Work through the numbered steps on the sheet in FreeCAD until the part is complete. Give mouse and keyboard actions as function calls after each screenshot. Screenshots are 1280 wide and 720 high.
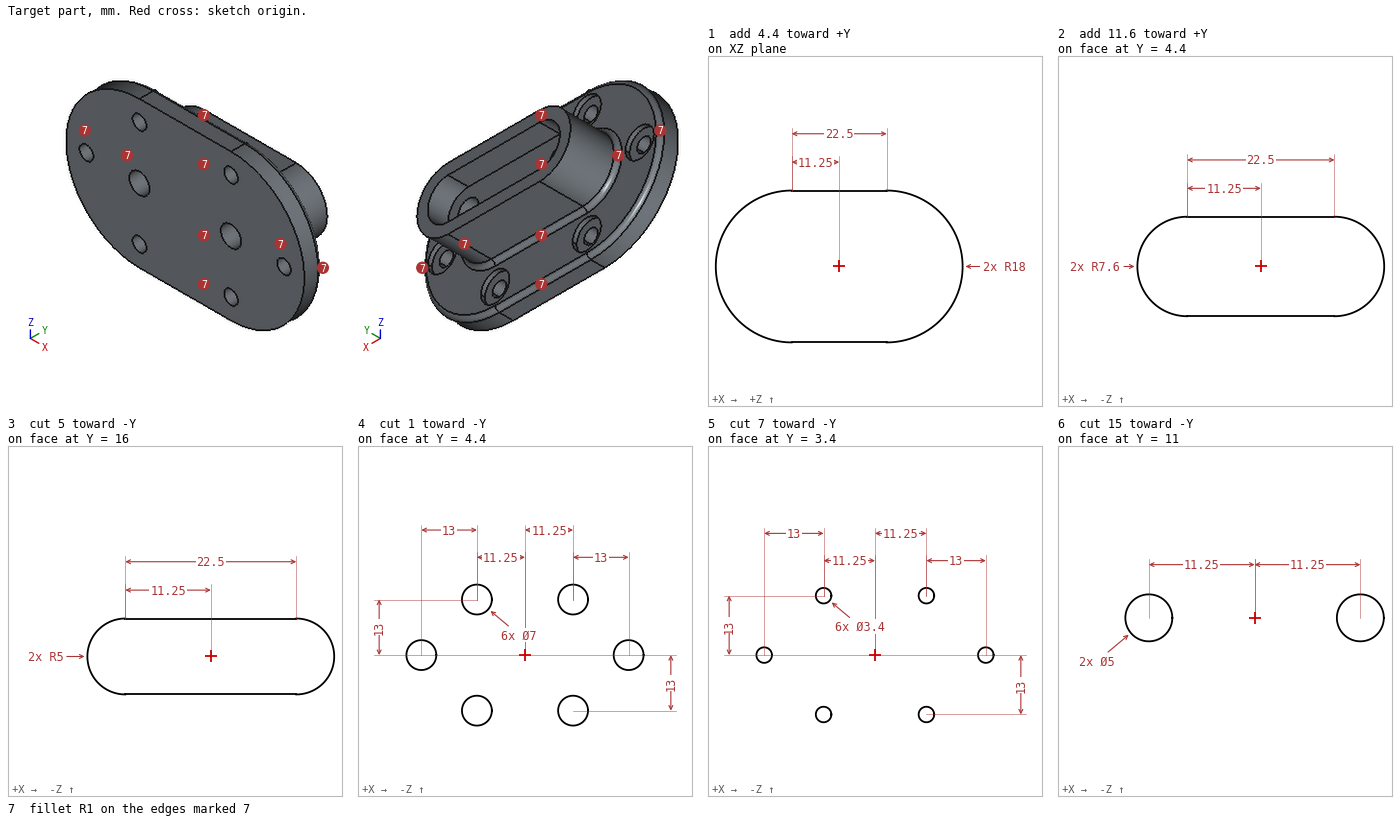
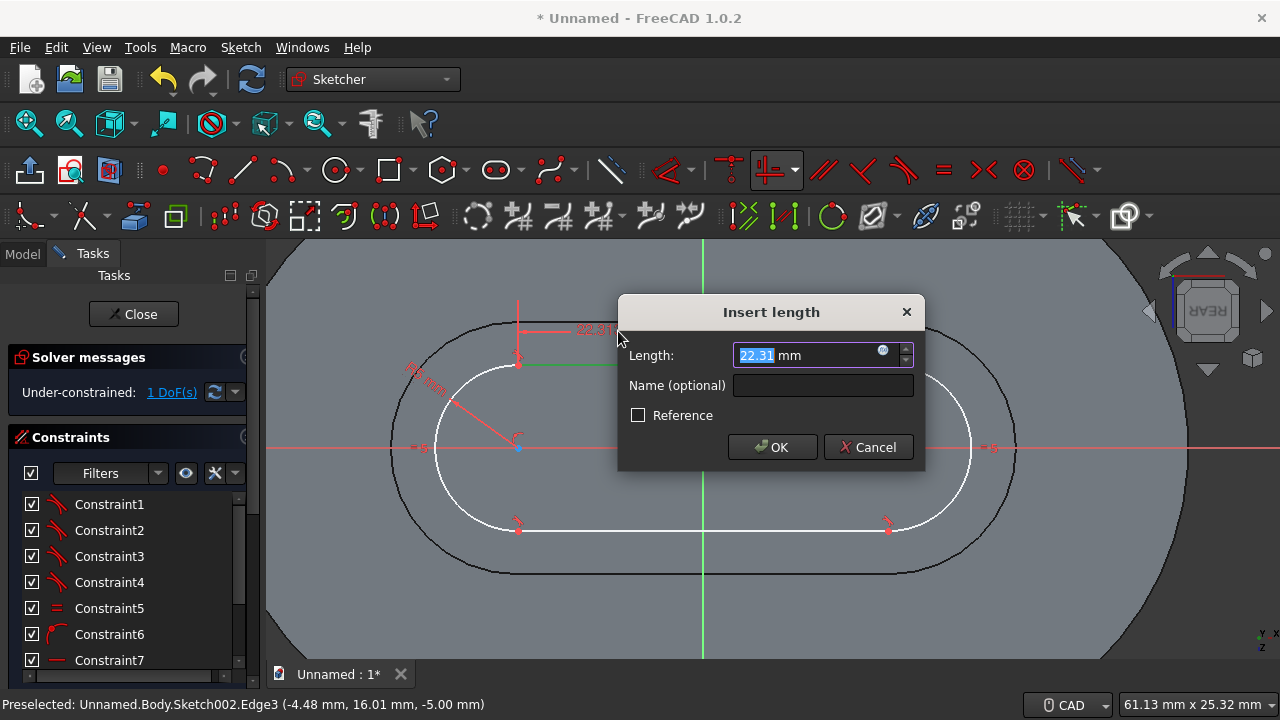
text(22.5)
key(Return)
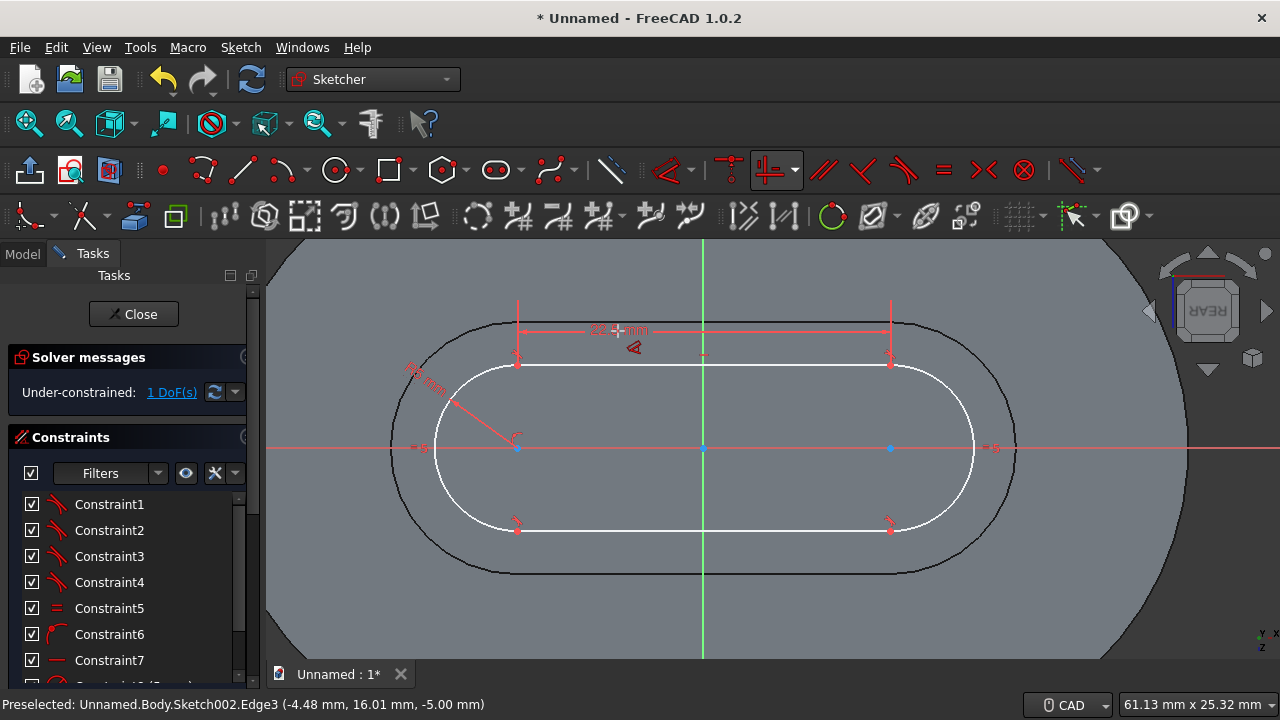
click(518, 365)
click(546, 331)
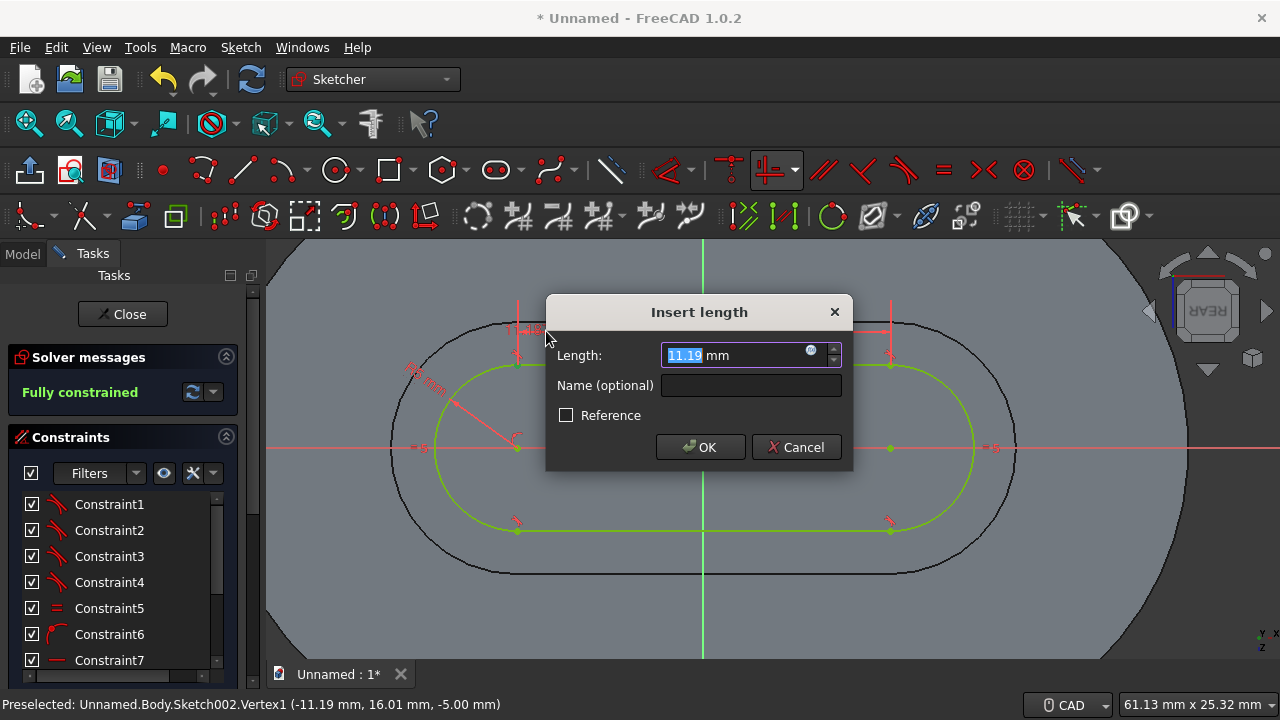
text(11.25)
key(Return)
key(Escape)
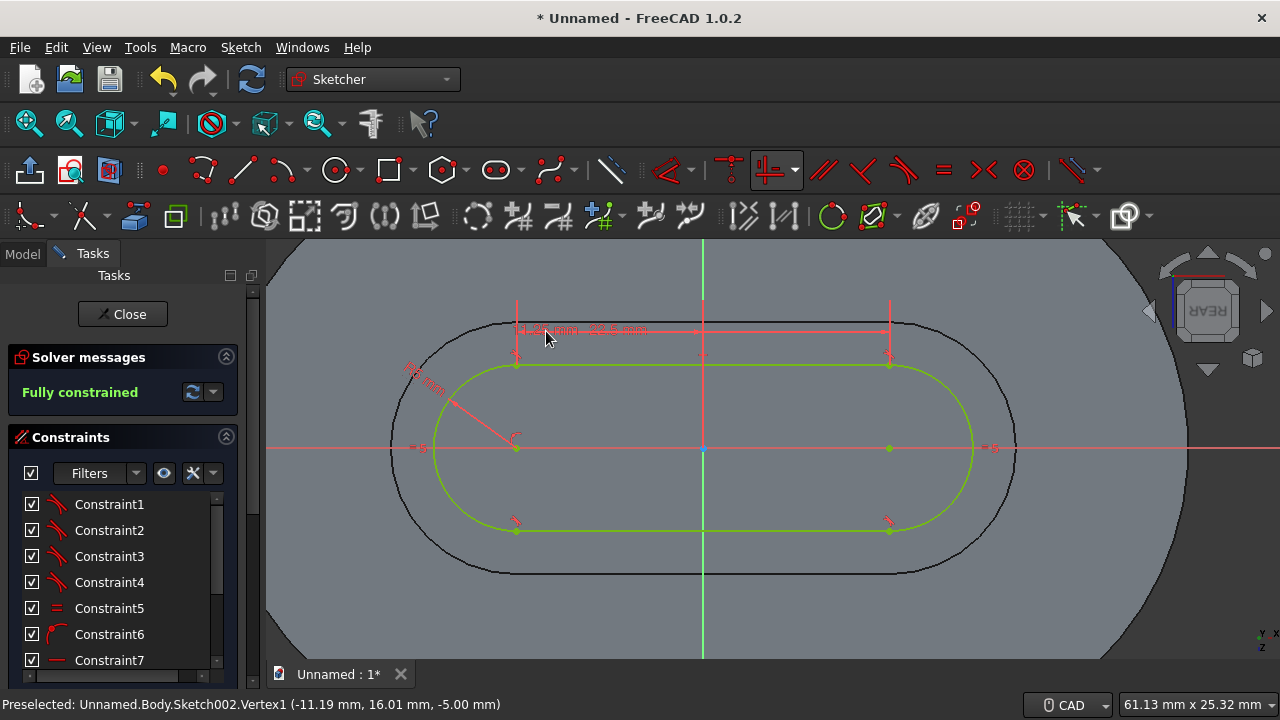
click(123, 314)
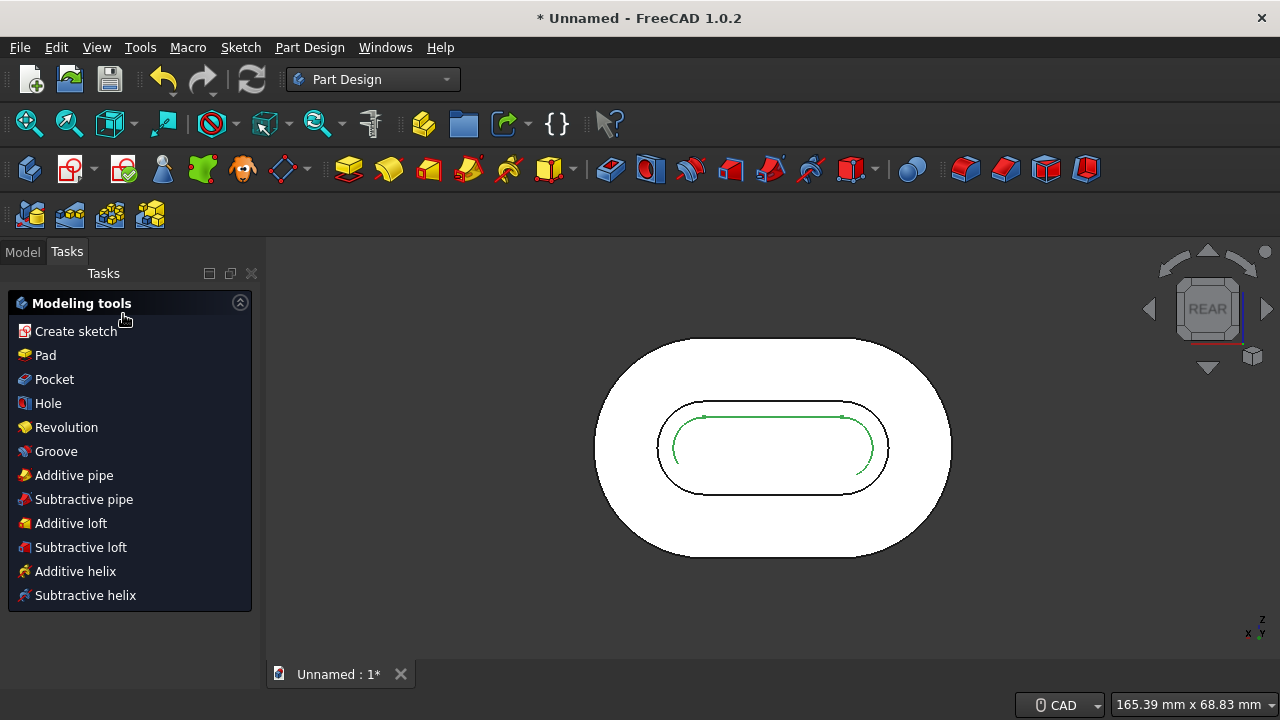
click(612, 170)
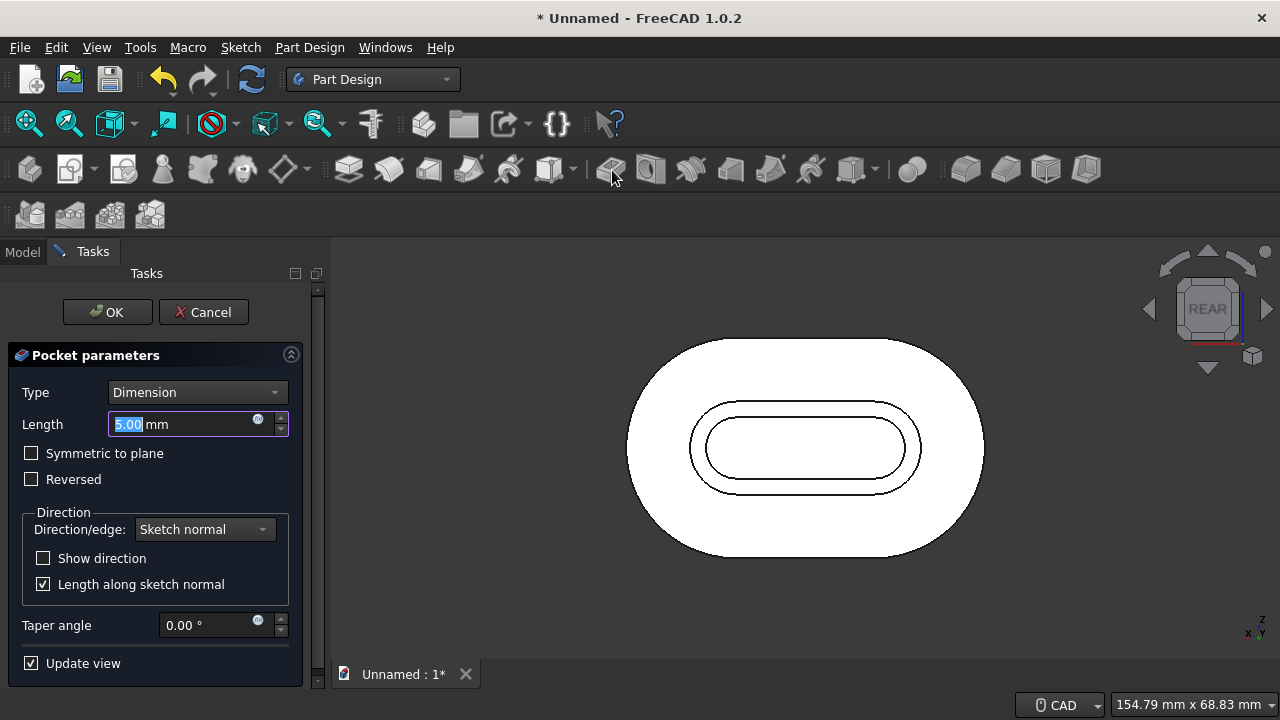
text(5)
key(Tab)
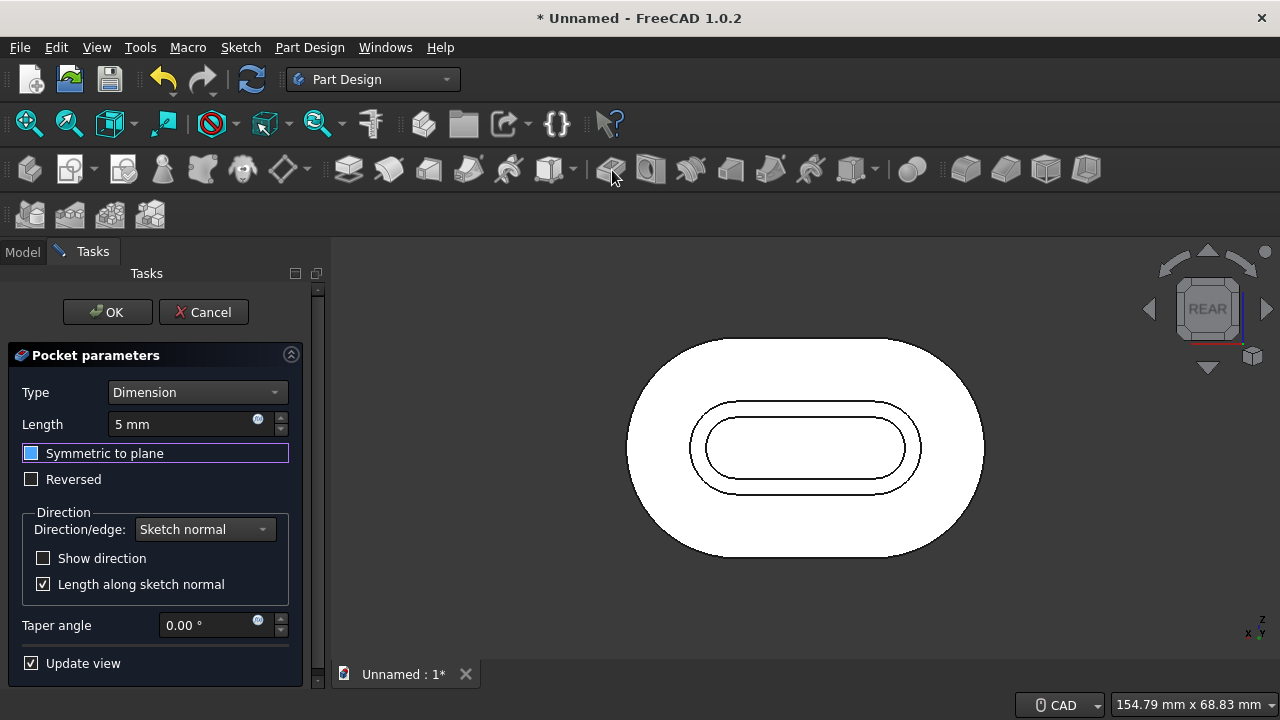
click(108, 312)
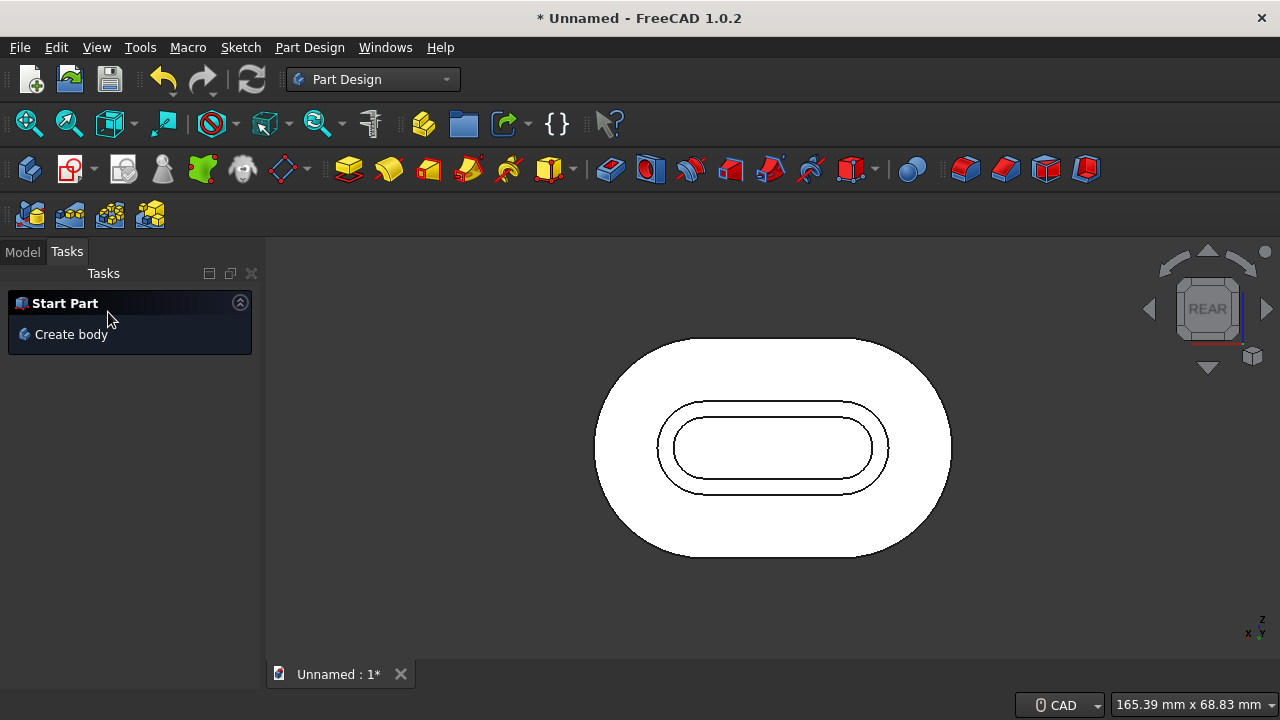
click(619, 447)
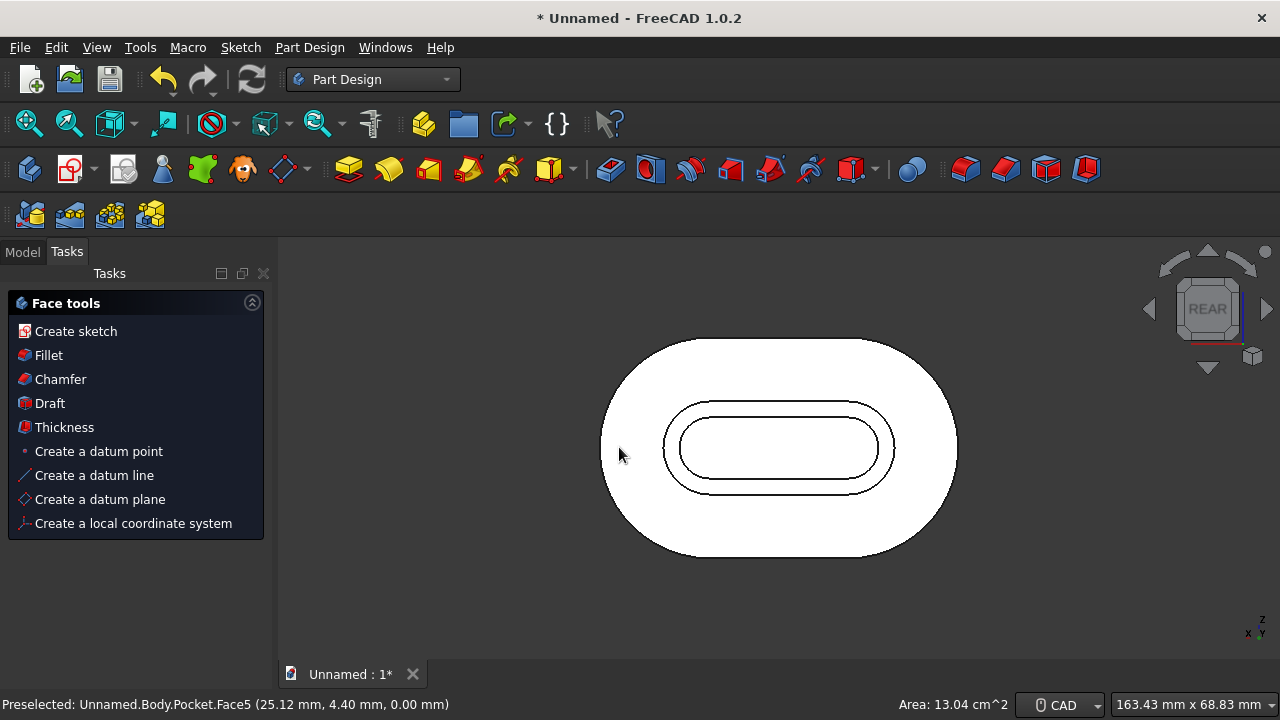
click(70, 170)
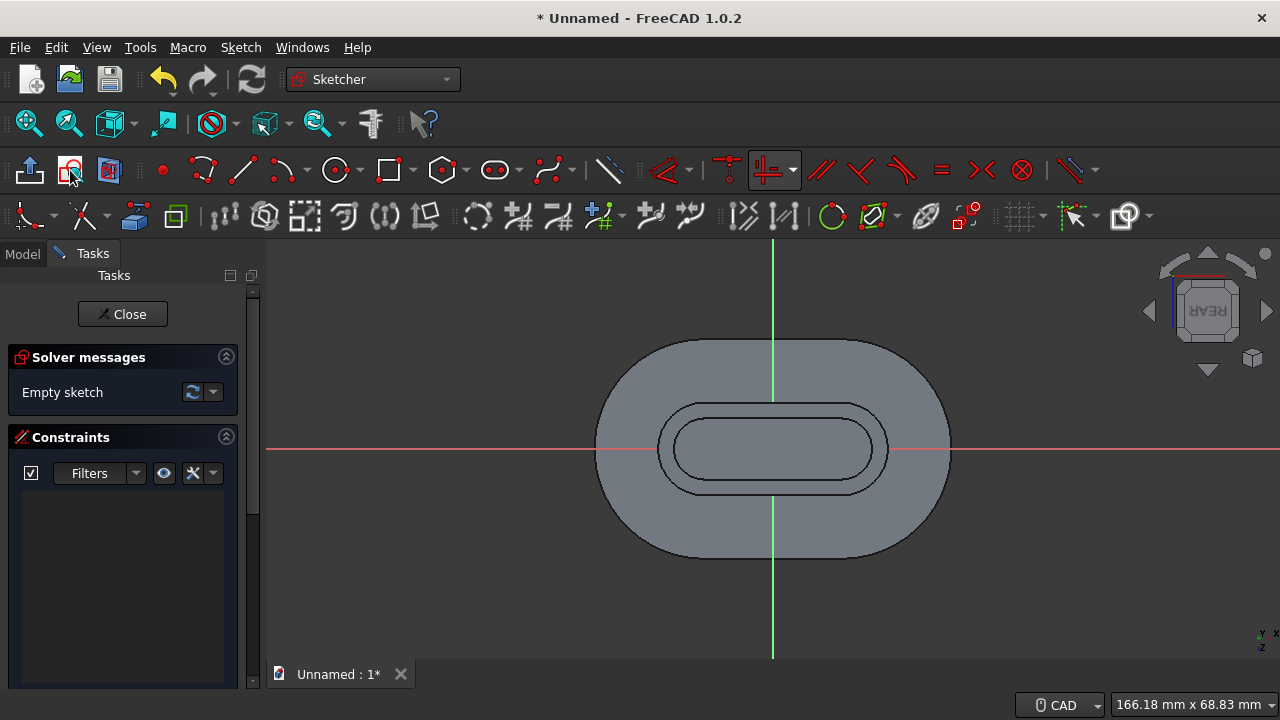
click(110, 170)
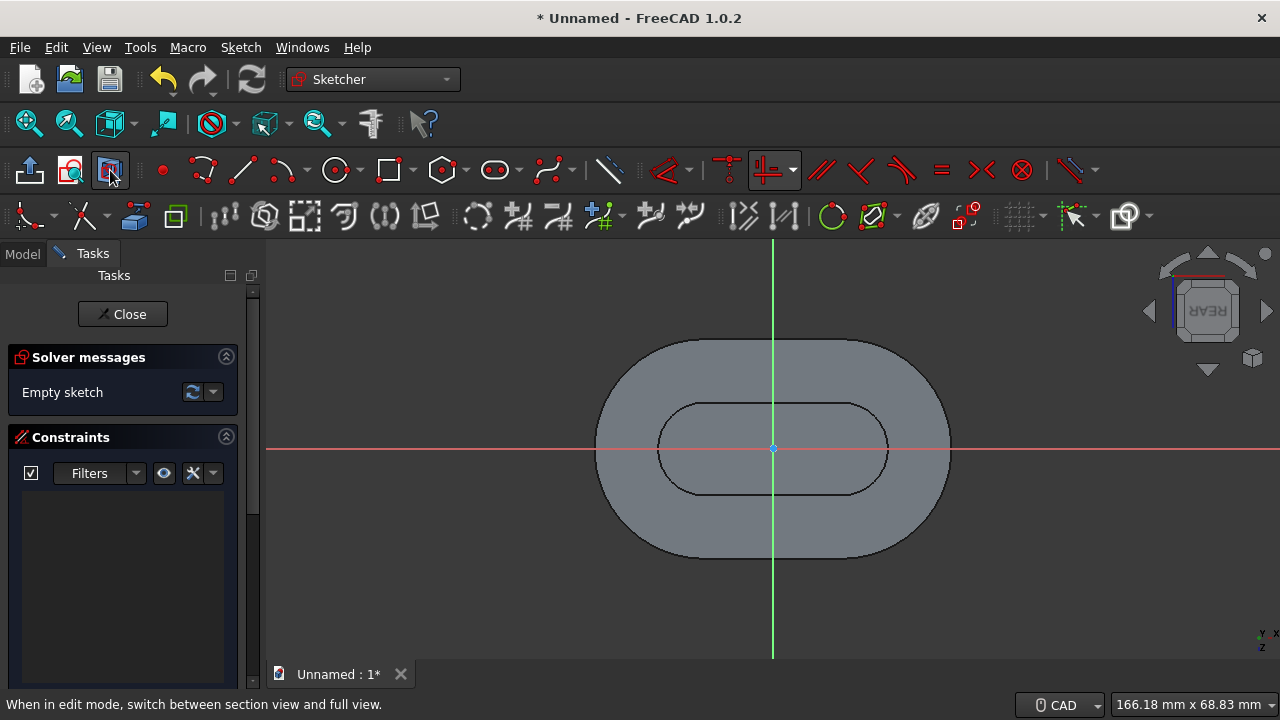
click(336, 170)